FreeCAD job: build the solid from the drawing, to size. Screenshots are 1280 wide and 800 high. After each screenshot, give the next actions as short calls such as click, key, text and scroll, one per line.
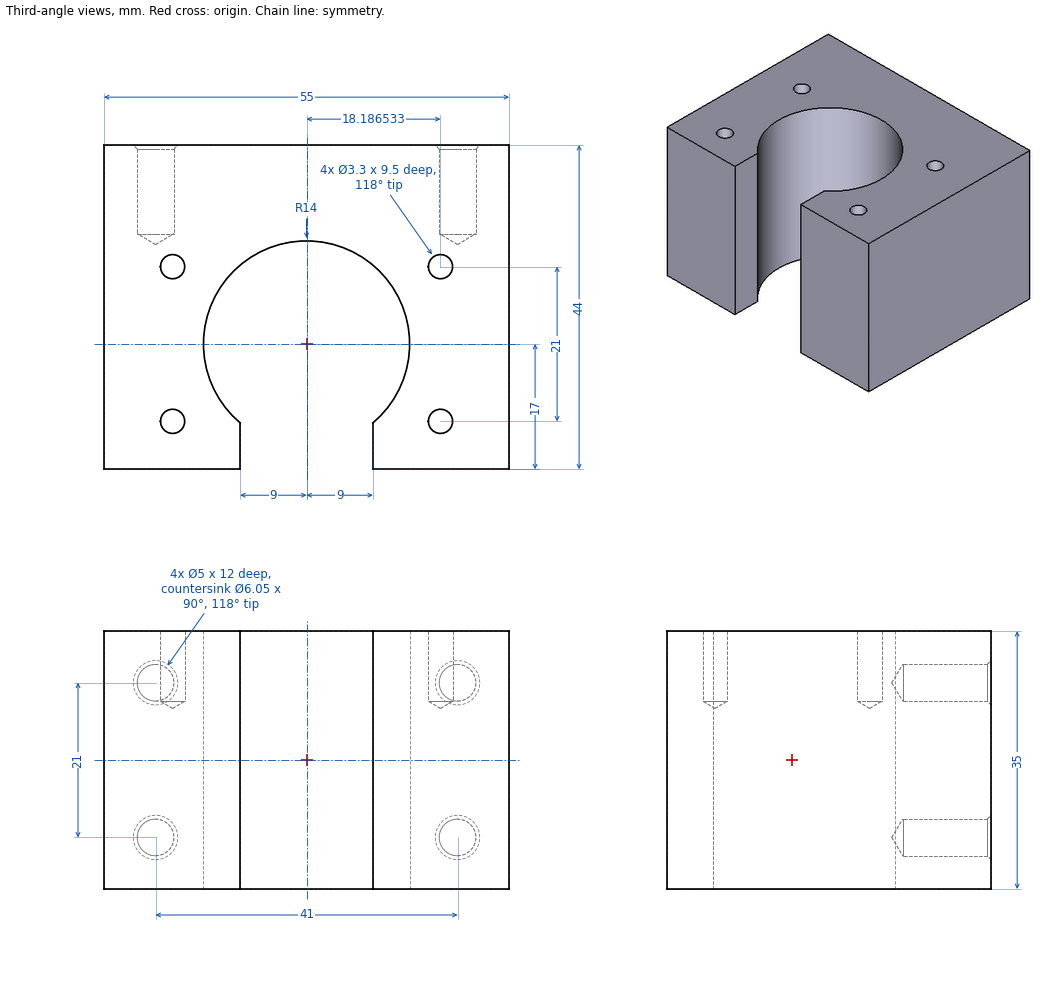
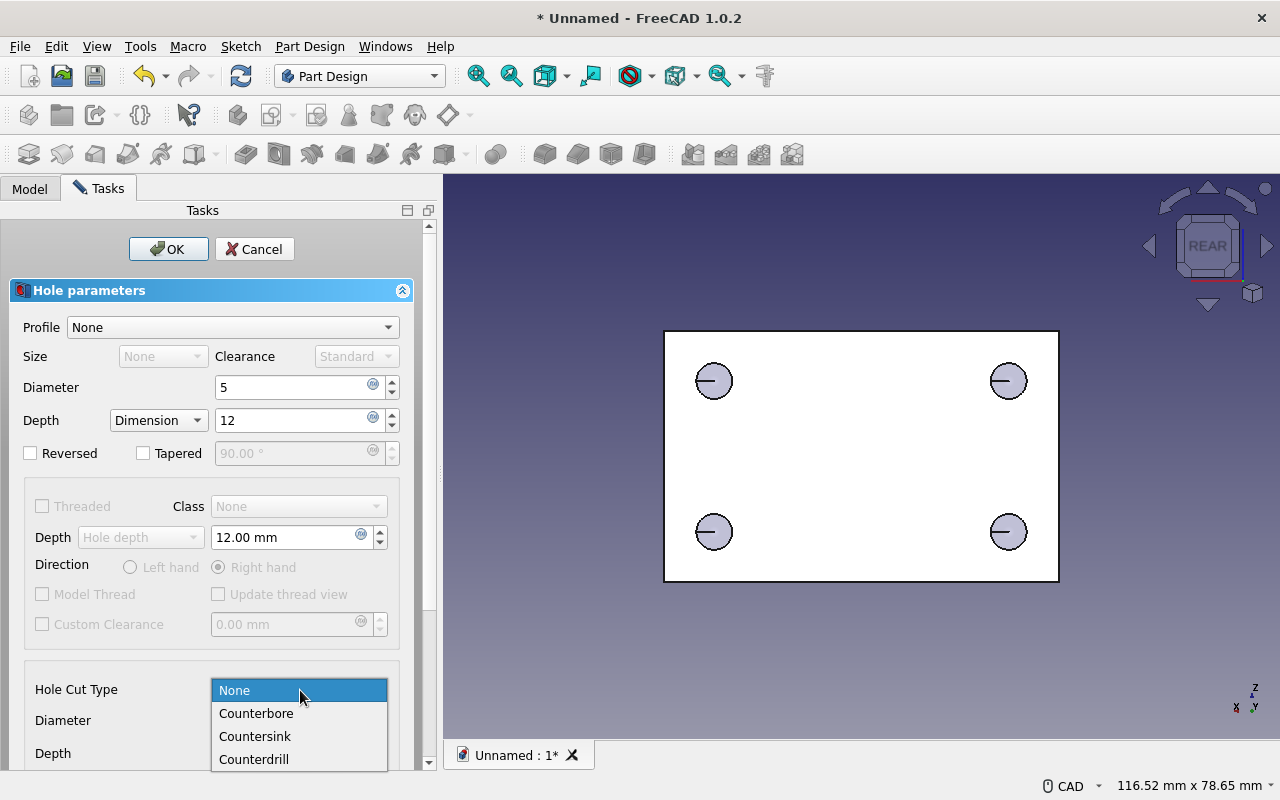
click(298, 736)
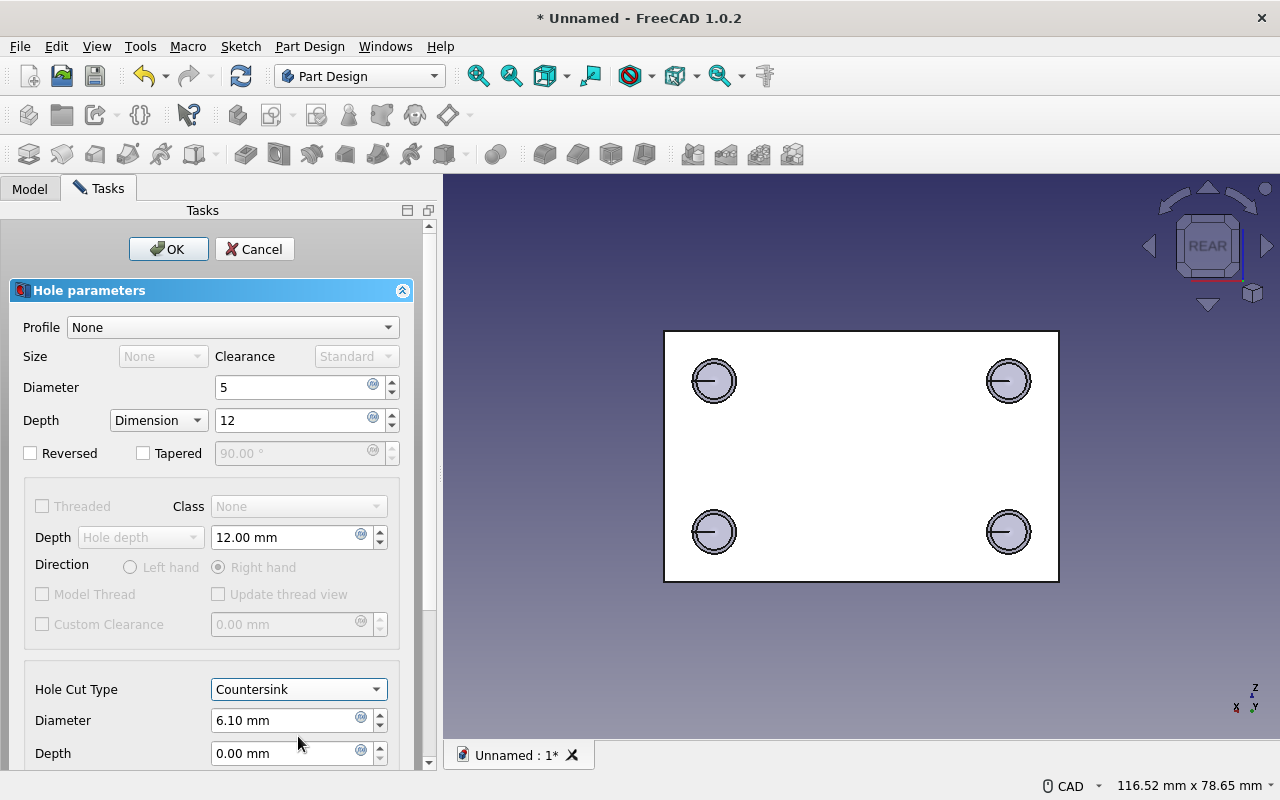
triple_click(292, 720)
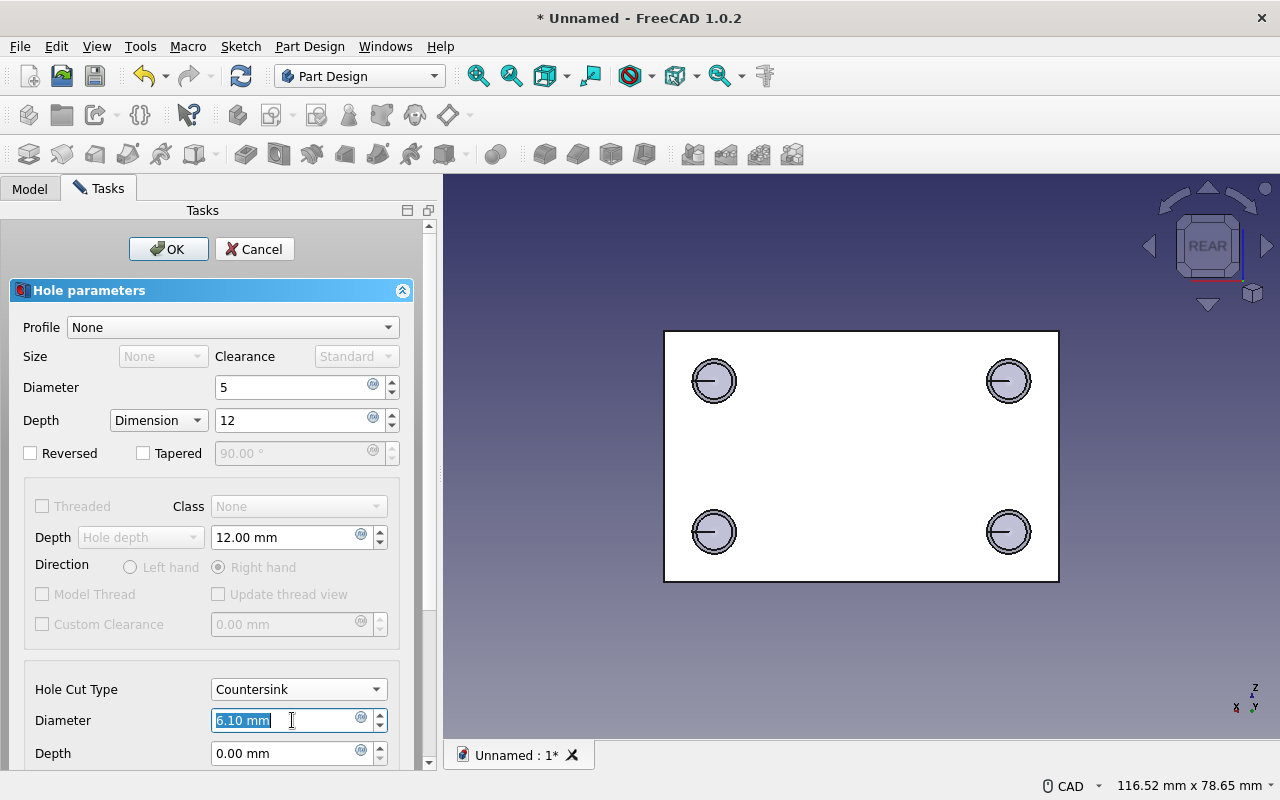
text(6.05)
key(Tab)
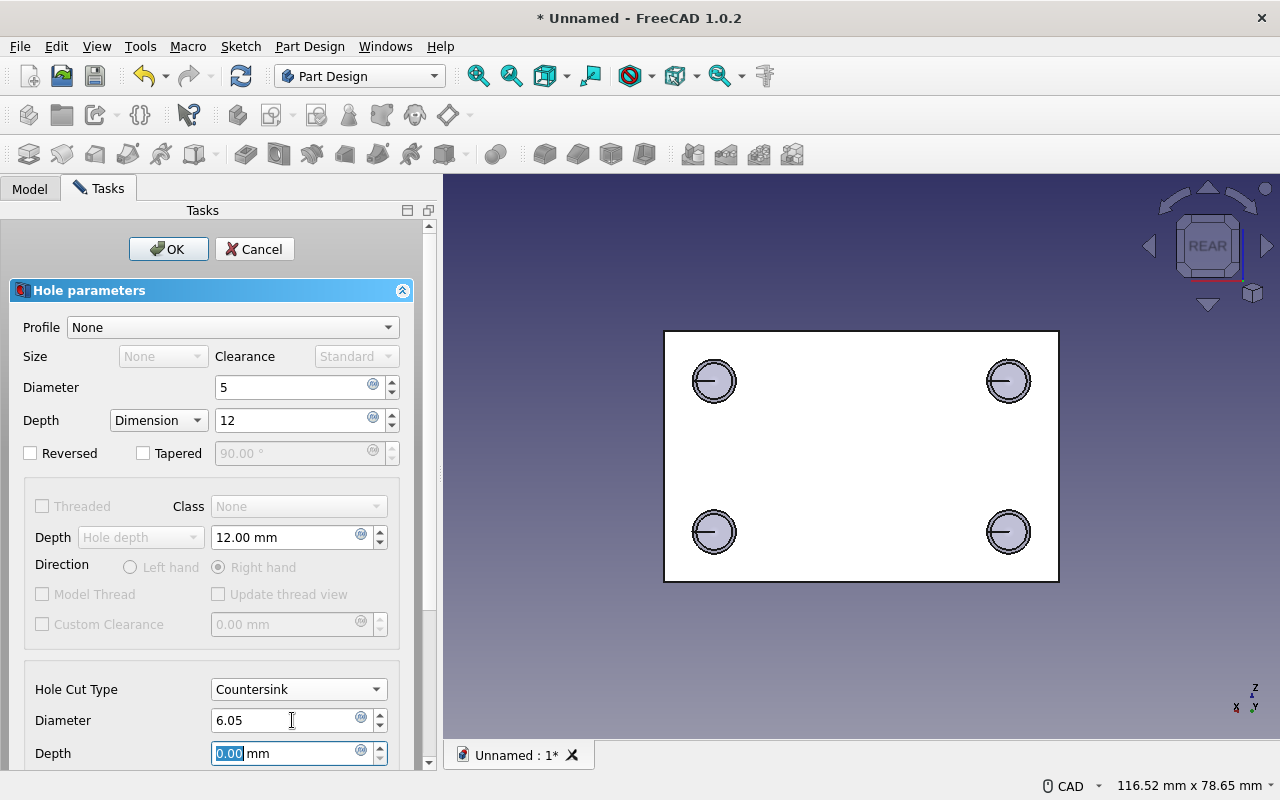
click(169, 249)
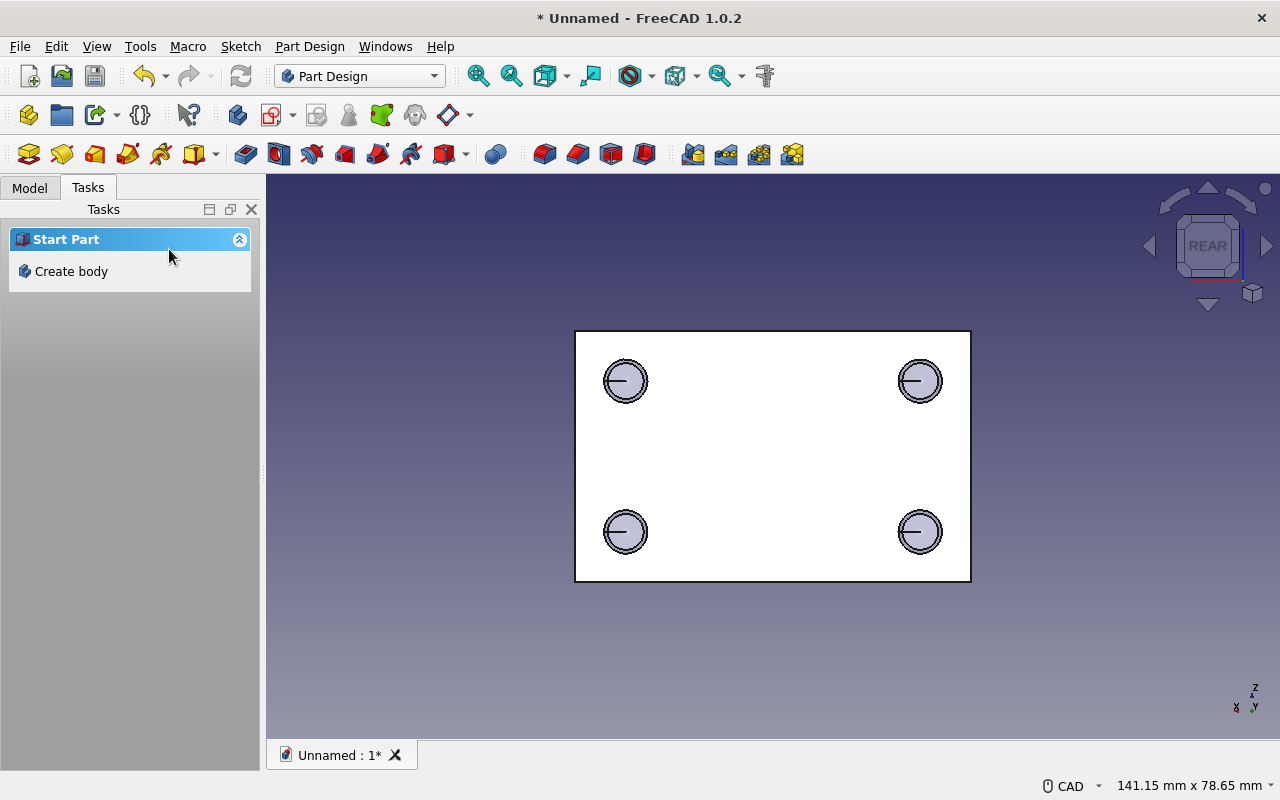
key(0)